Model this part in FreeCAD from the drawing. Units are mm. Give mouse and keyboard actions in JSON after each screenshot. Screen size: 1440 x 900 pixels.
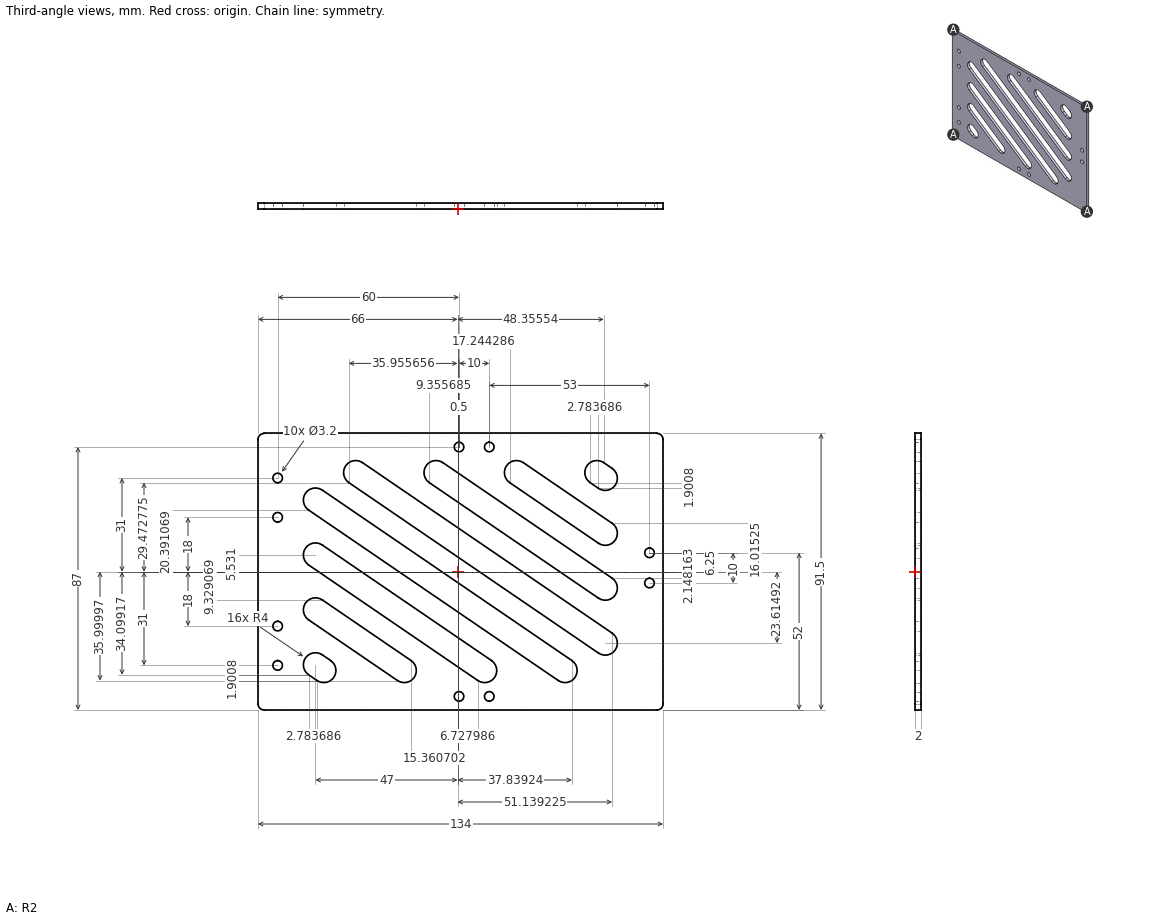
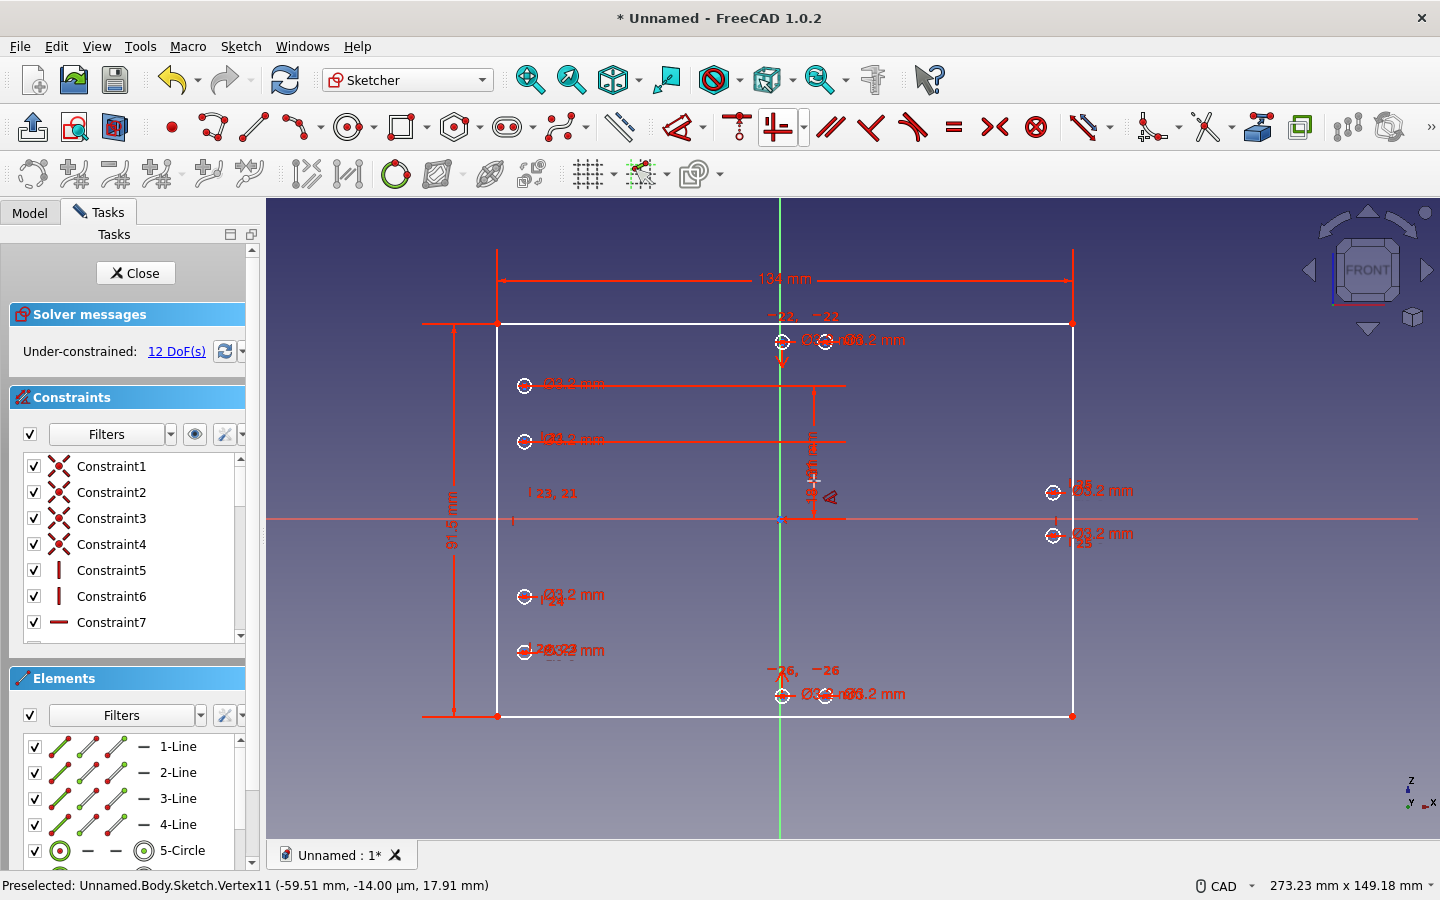
{"action": "left_click", "coordinate": [525, 597]}
{"action": "left_click", "coordinate": [814, 558]}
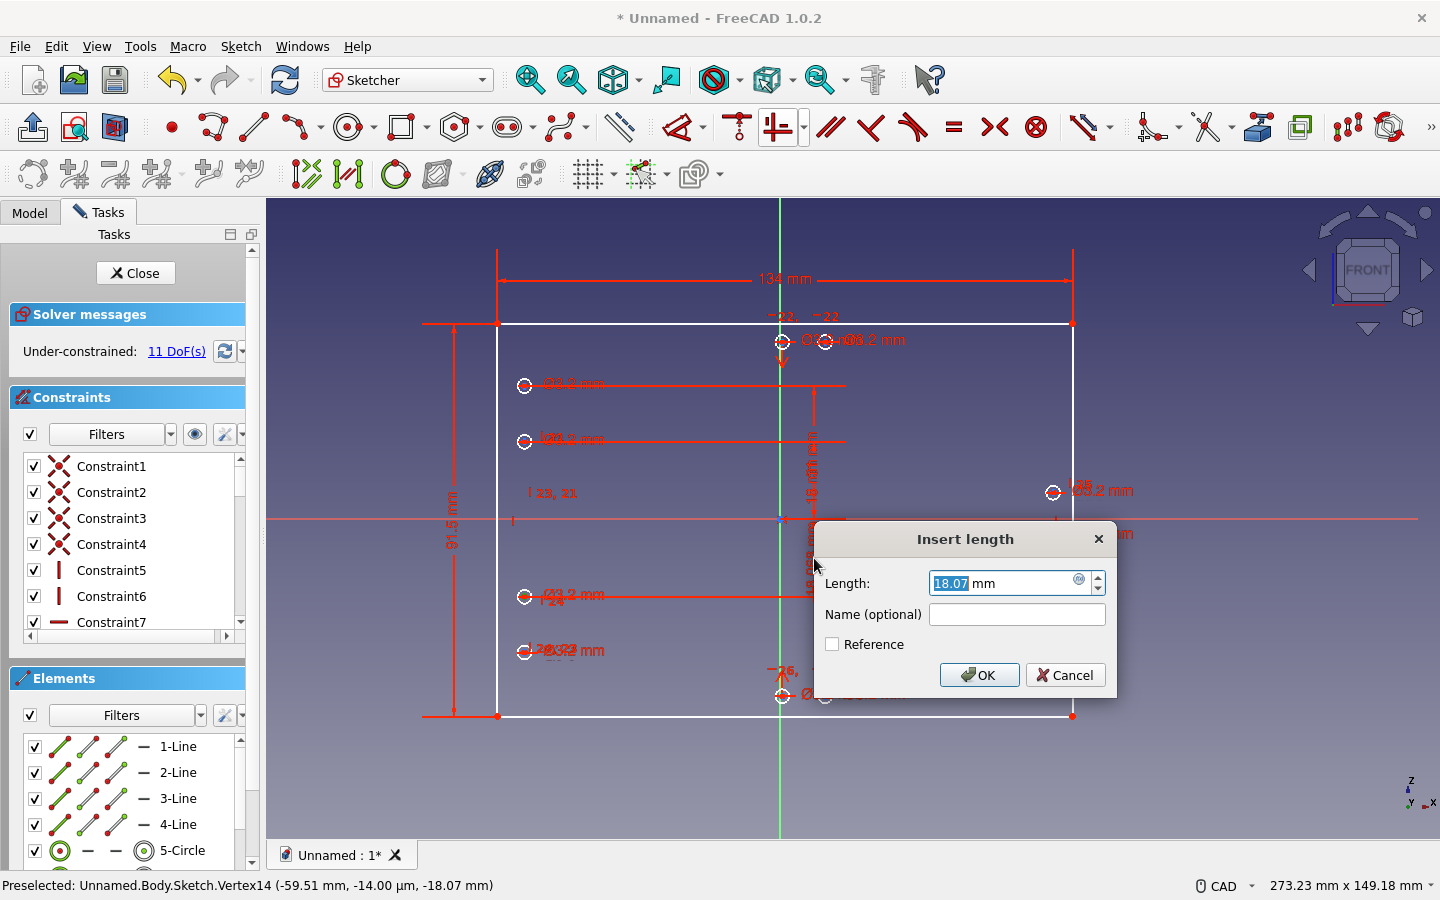
{"action": "type", "text": "18"}
{"action": "key", "text": "Return"}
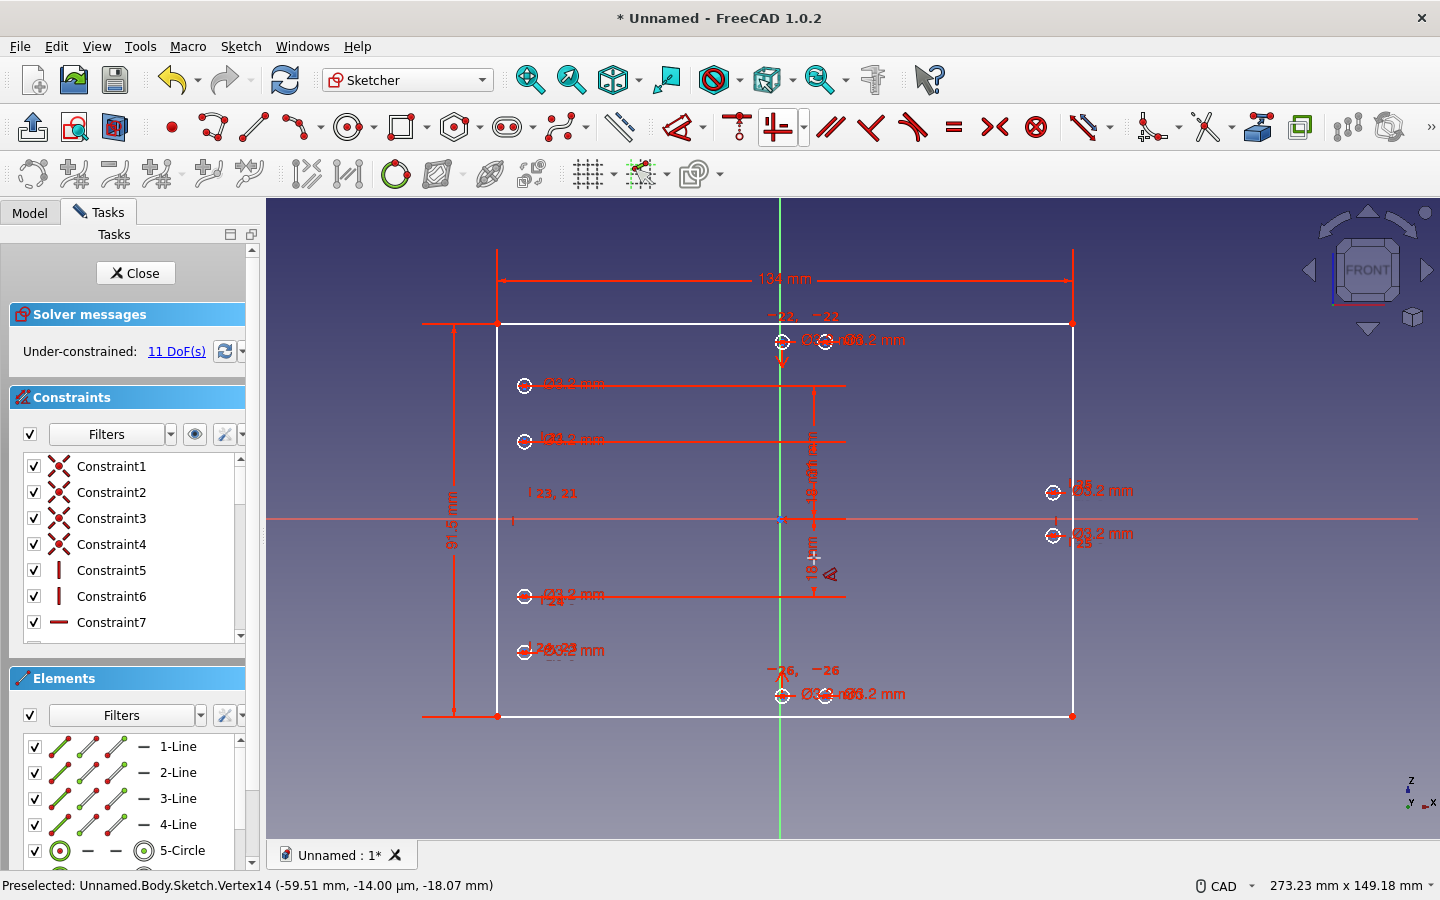
{"action": "left_click", "coordinate": [525, 653]}
{"action": "left_click", "coordinate": [814, 586]}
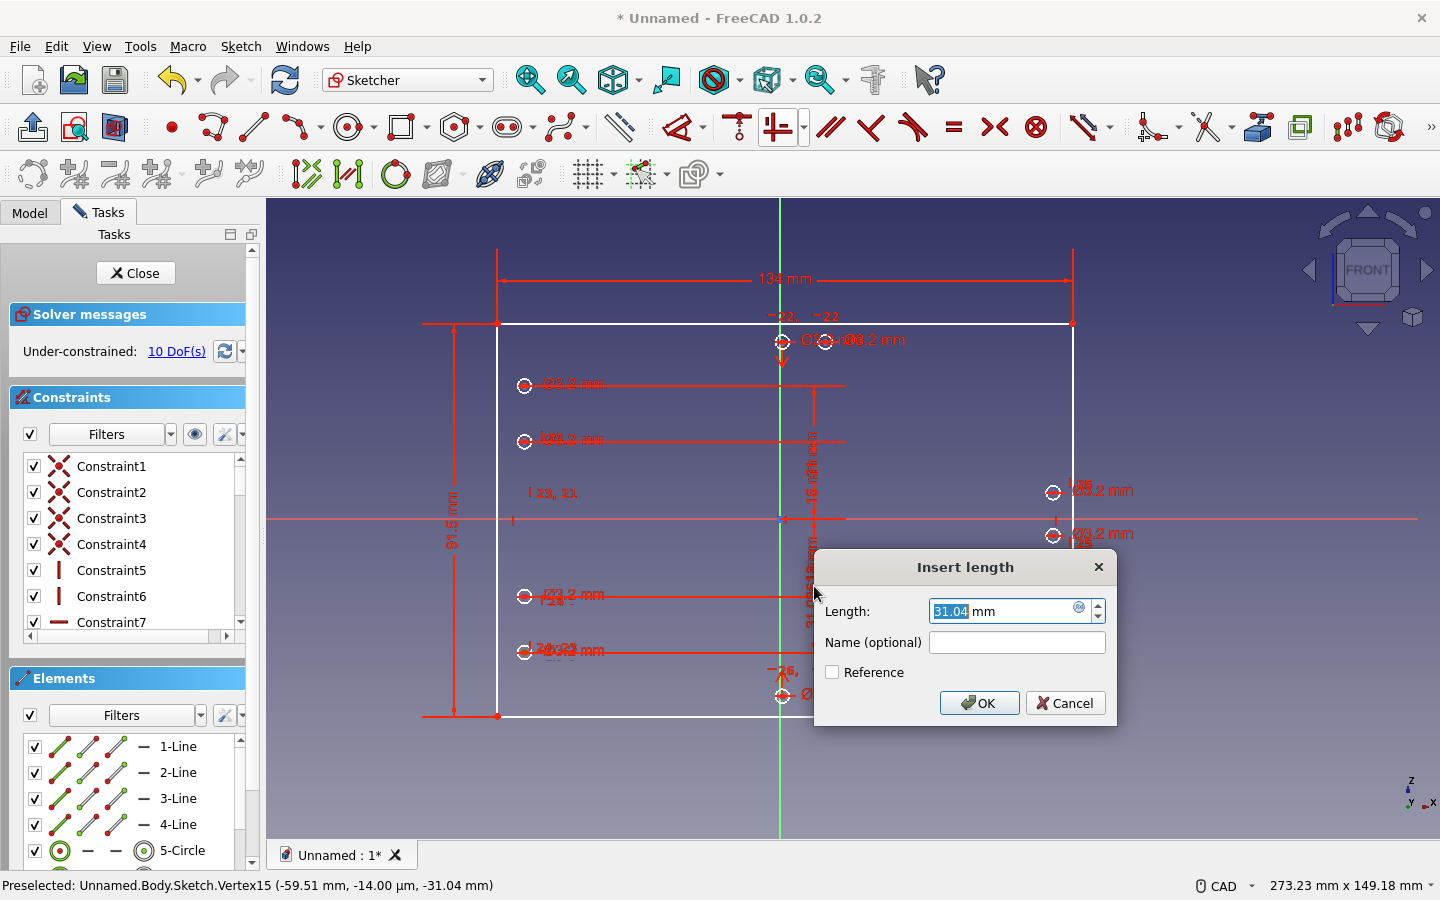
{"action": "type", "text": "31"}
{"action": "key", "text": "Return"}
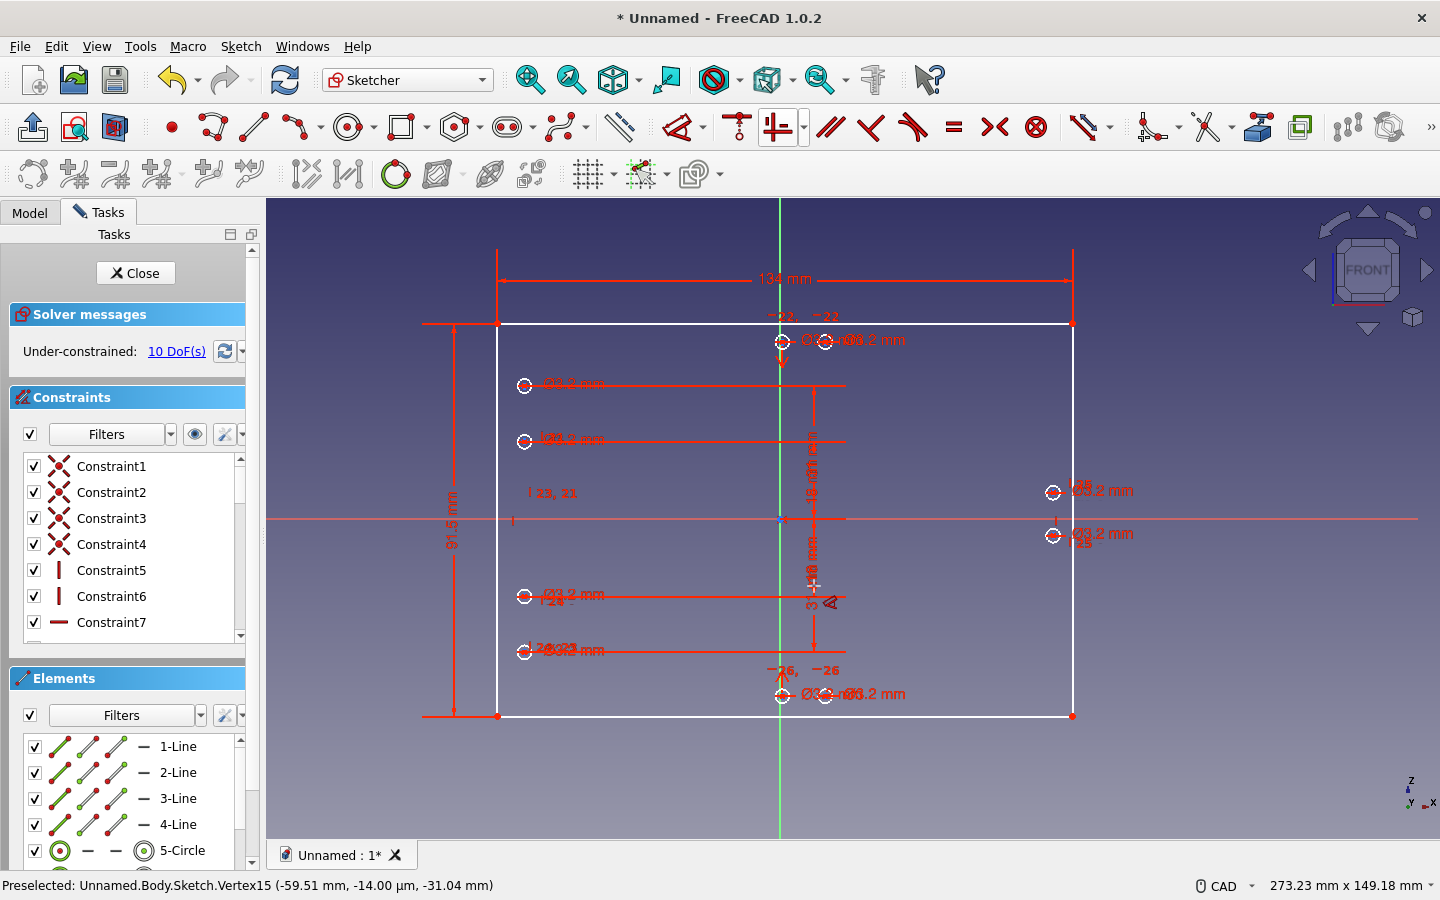
{"action": "left_click", "coordinate": [497, 324]}
{"action": "left_click", "coordinate": [639, 290]}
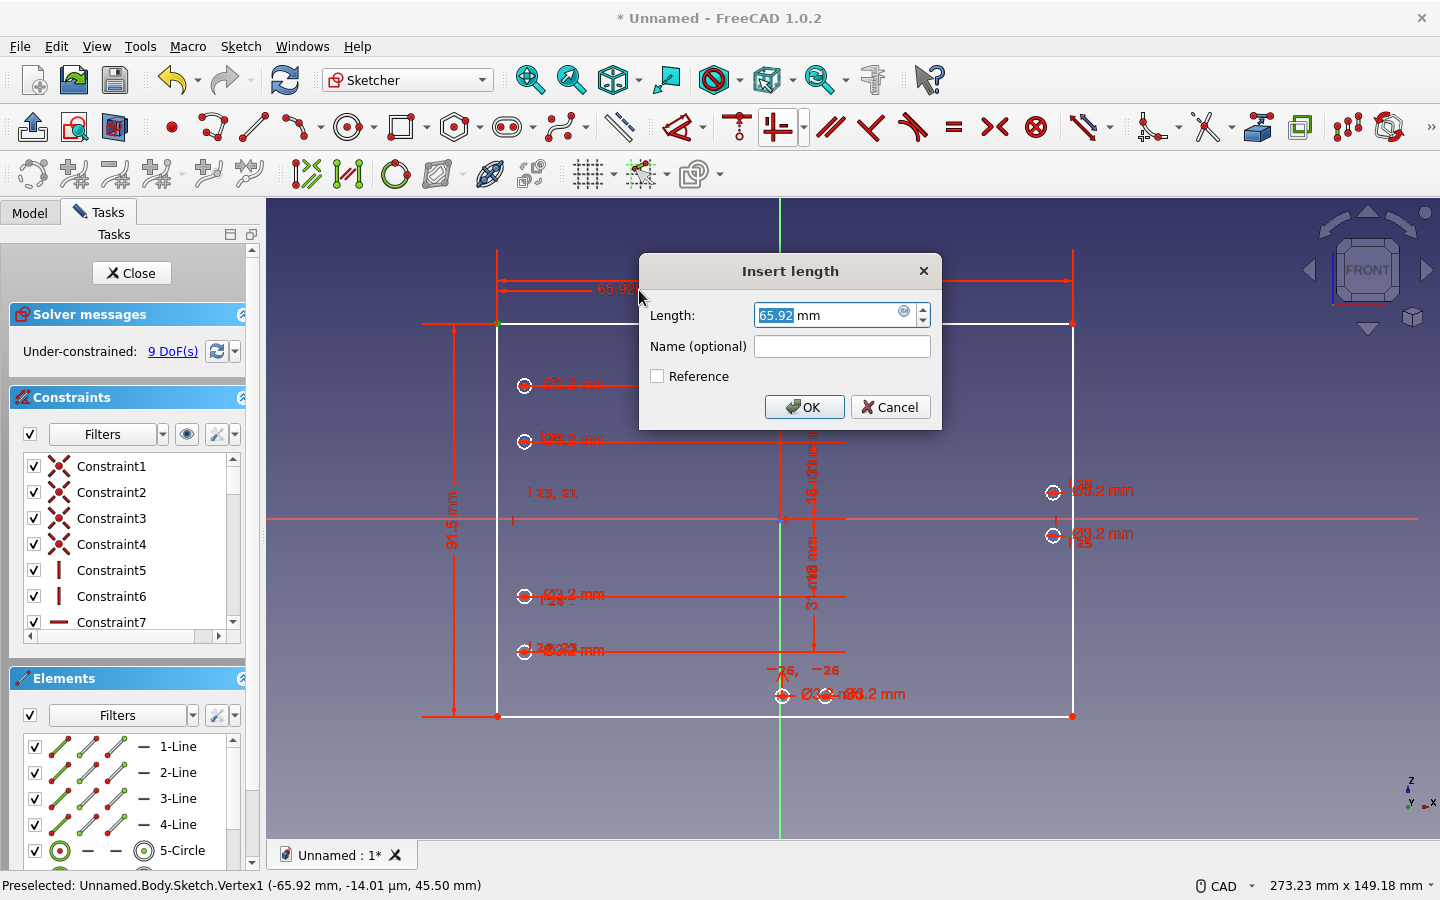
{"action": "type", "text": "66"}
{"action": "key", "text": "Return"}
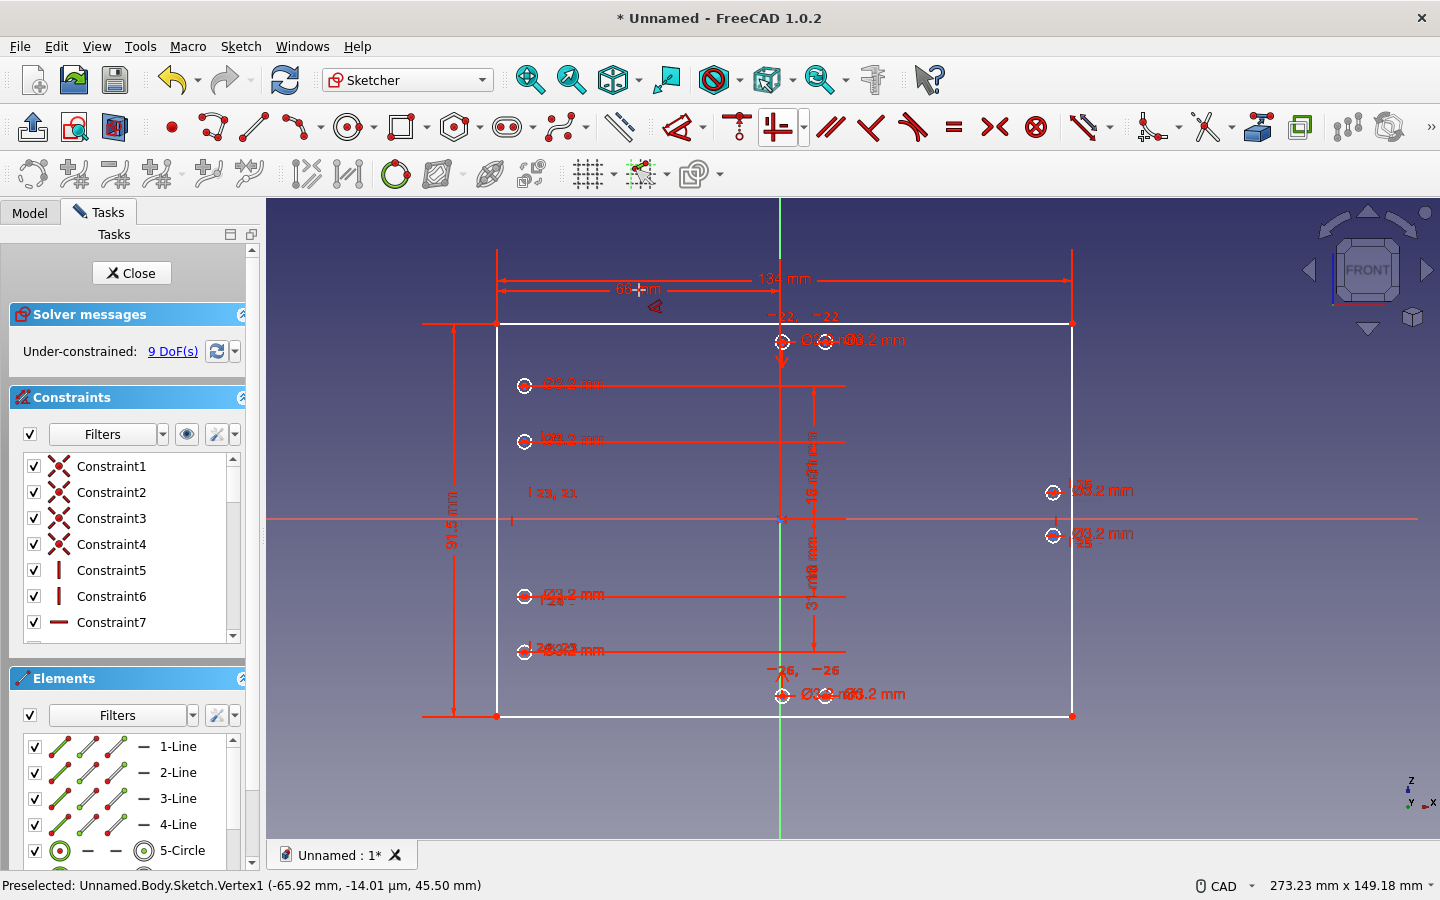
{"action": "scroll", "coordinate": [782, 342], "scroll_direction": "up", "scroll_amount": 15}